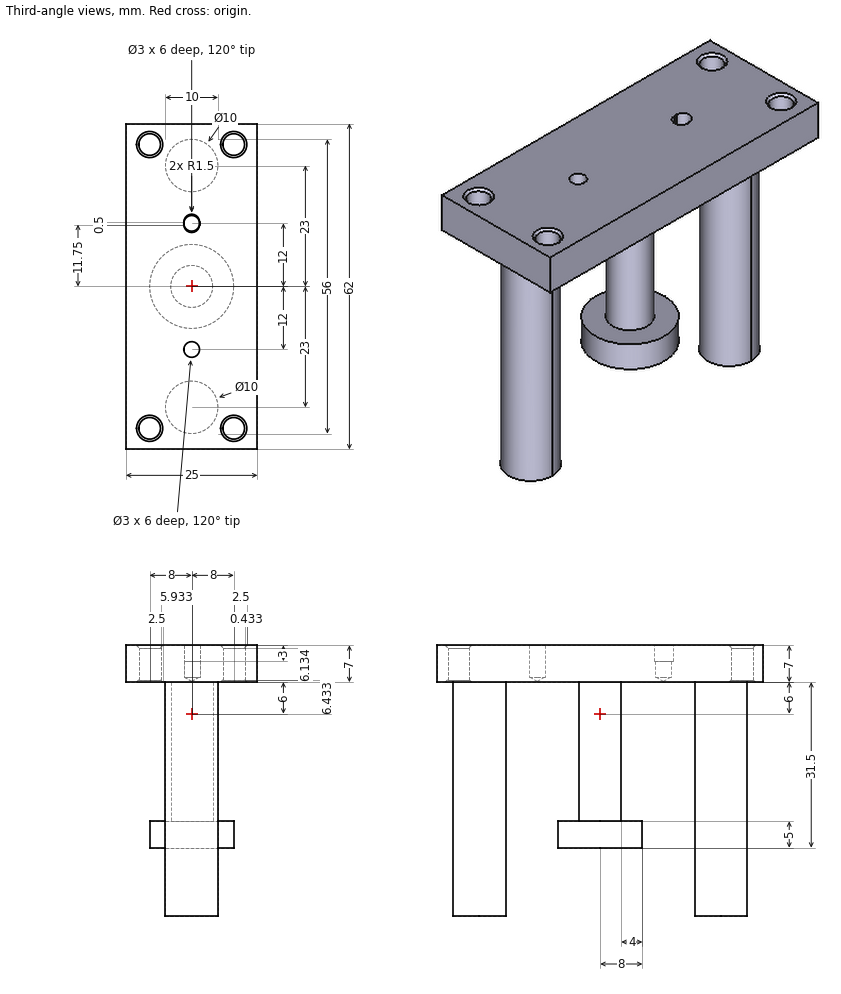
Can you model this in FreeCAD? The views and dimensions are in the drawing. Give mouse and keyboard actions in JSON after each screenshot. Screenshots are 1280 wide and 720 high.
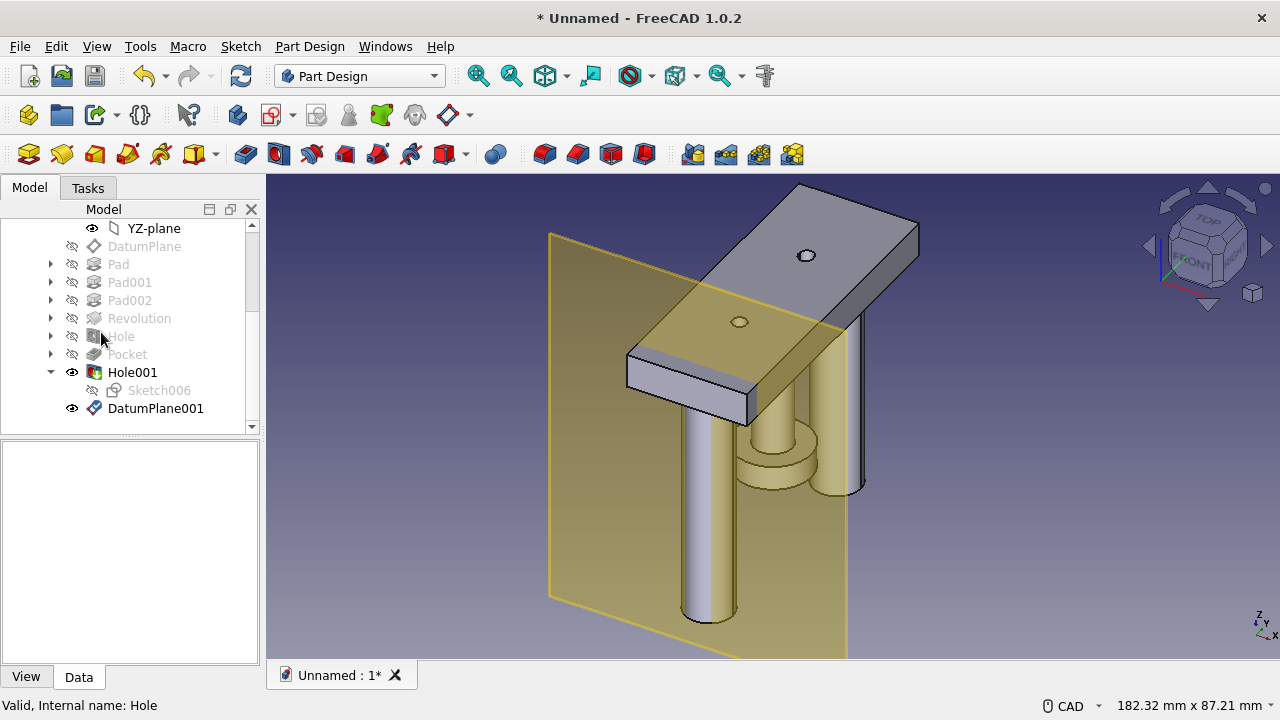
{"action": "left_click", "coordinate": [117, 408]}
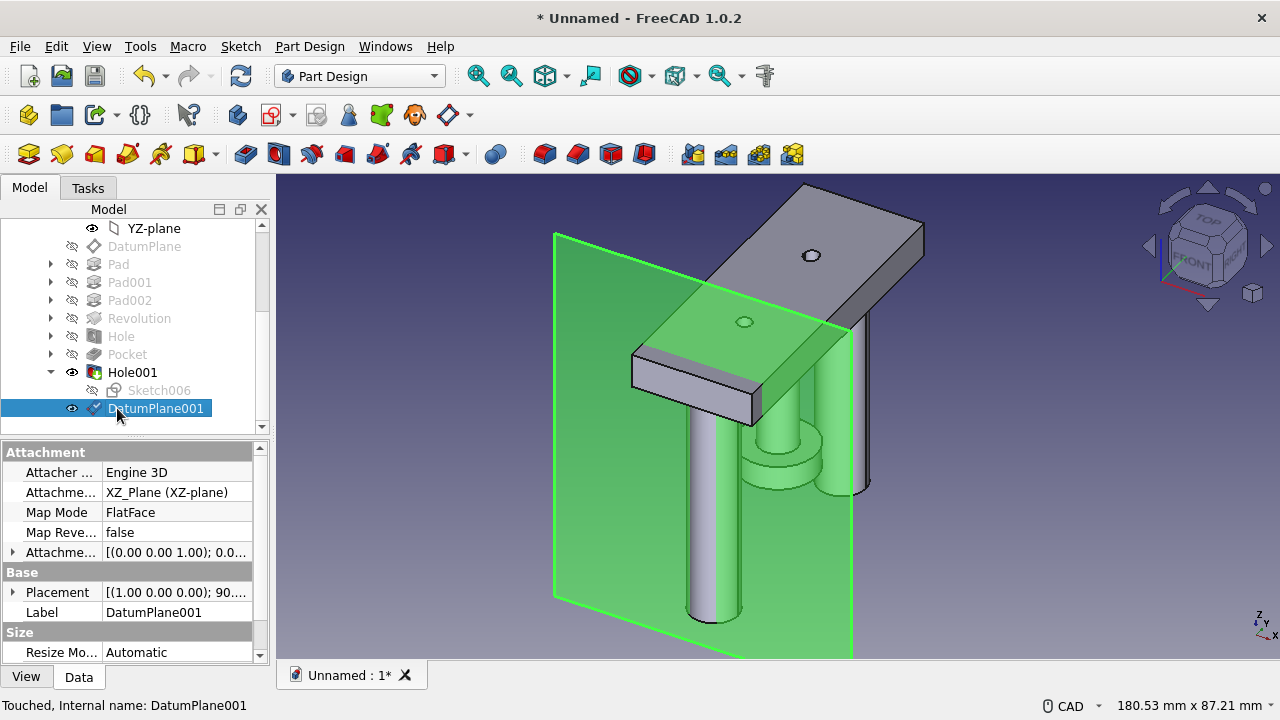
{"action": "left_click", "coordinate": [270, 116]}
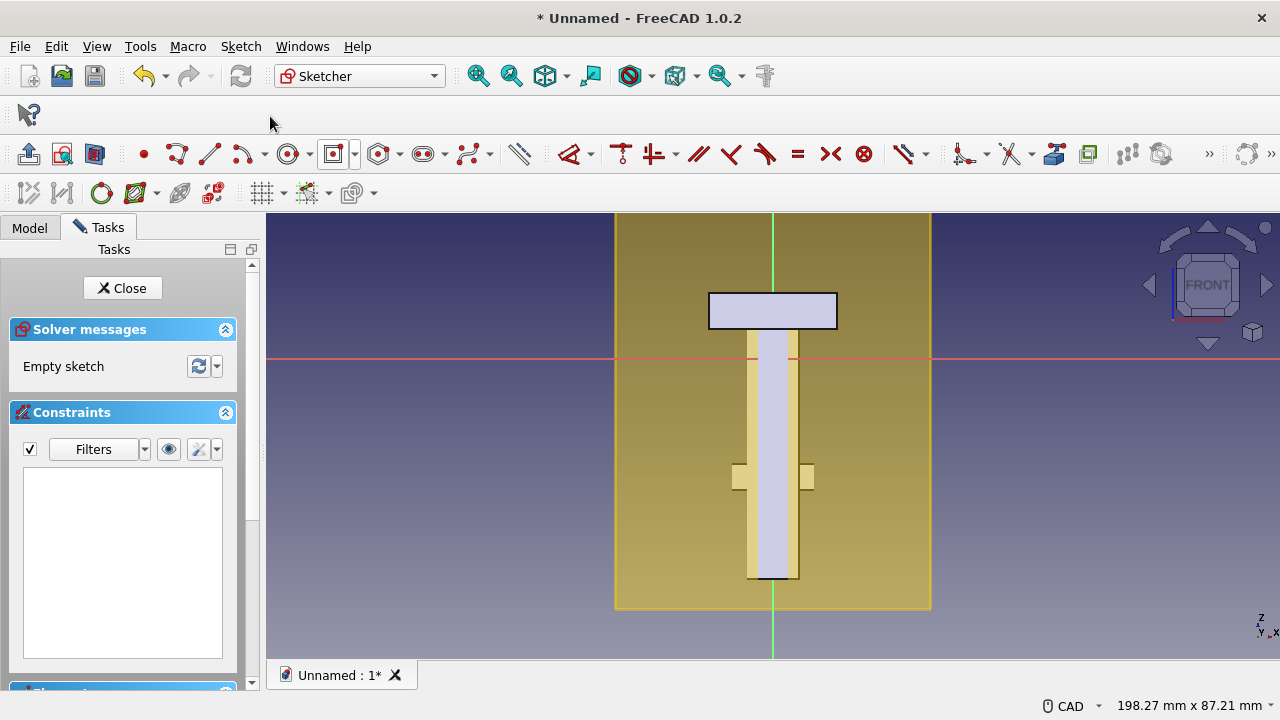
{"action": "left_click", "coordinate": [95, 154]}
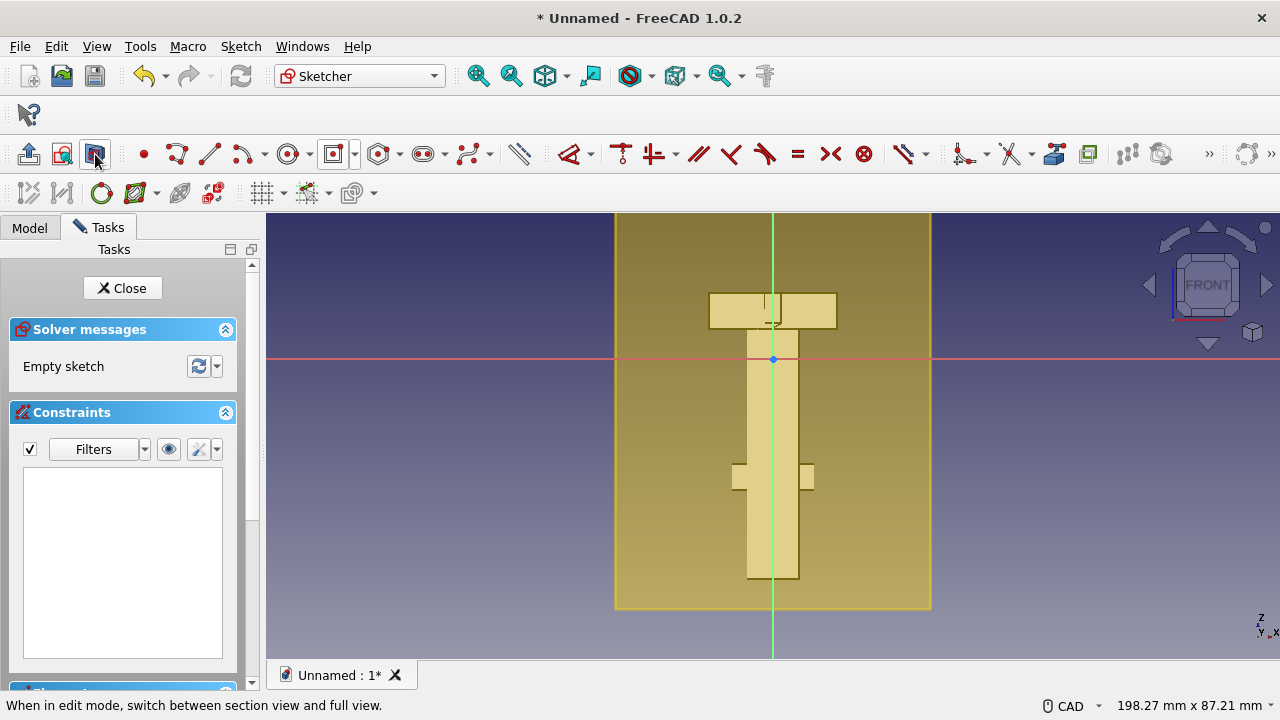
{"action": "scroll", "coordinate": [831, 290], "scroll_direction": "up", "scroll_amount": 7}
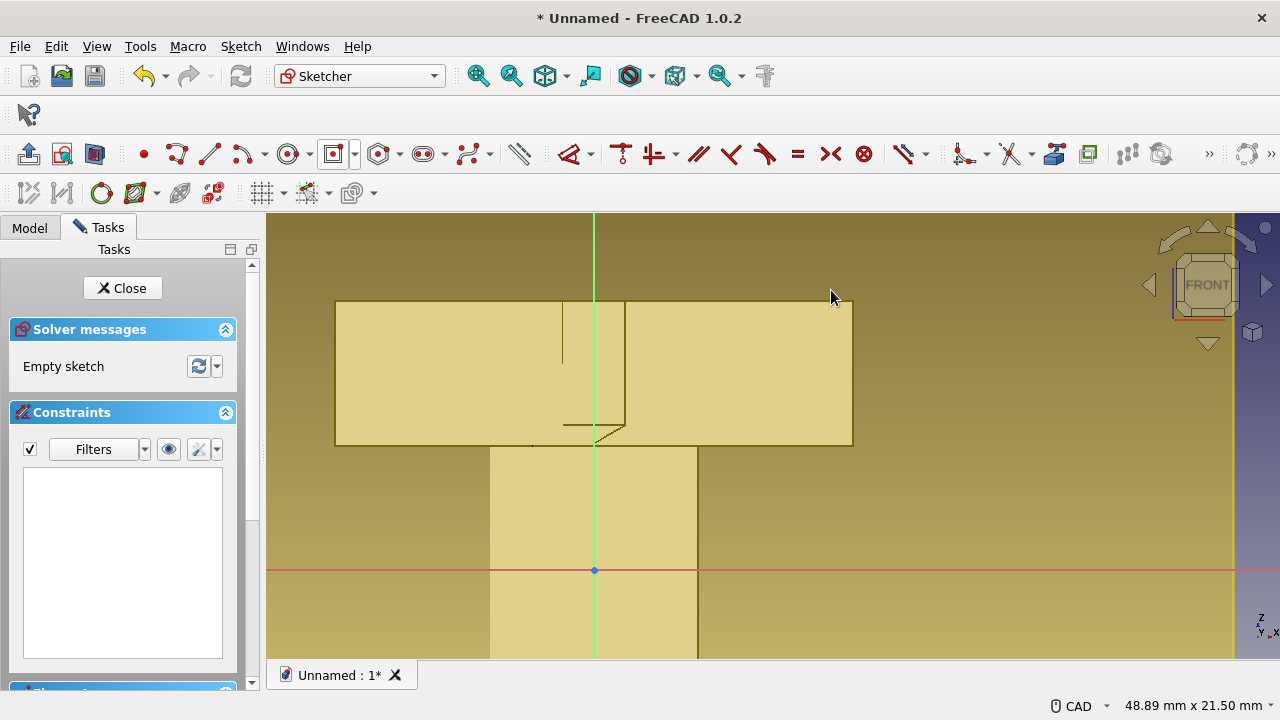
{"action": "left_click", "coordinate": [177, 154]}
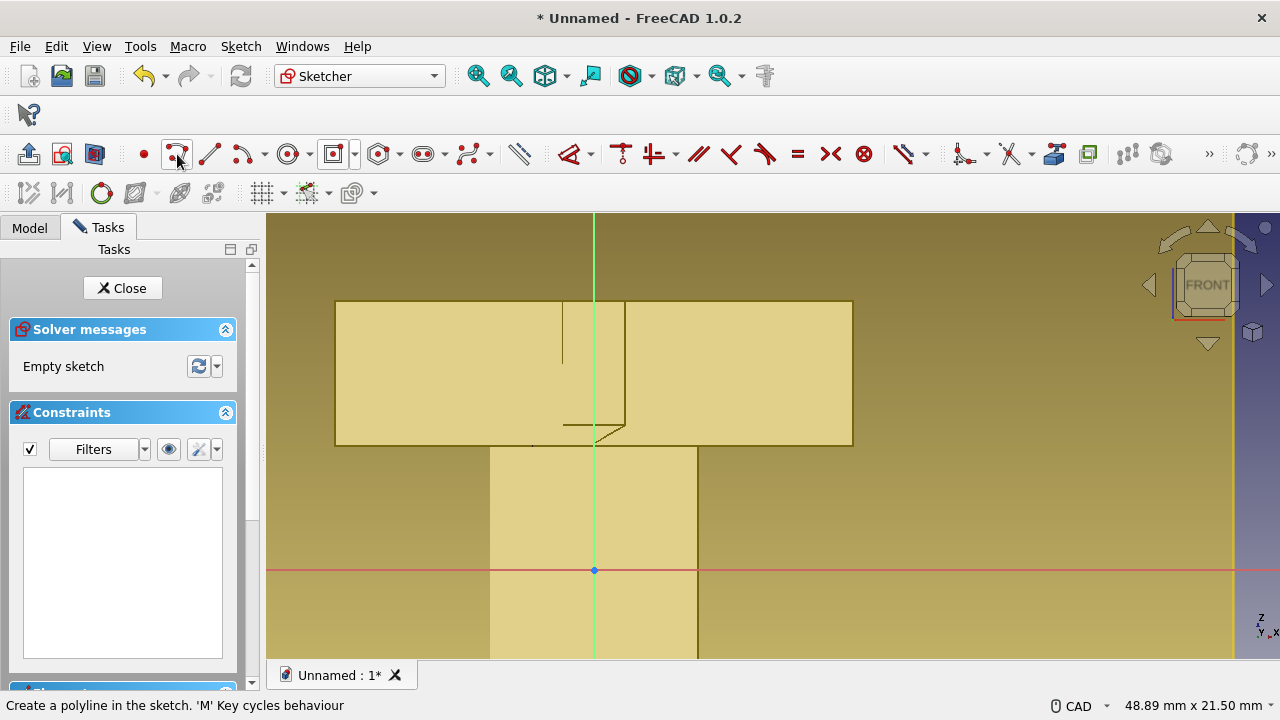
{"action": "left_click", "coordinate": [760, 446]}
{"action": "left_click", "coordinate": [760, 301]}
{"action": "left_click", "coordinate": [812, 301]}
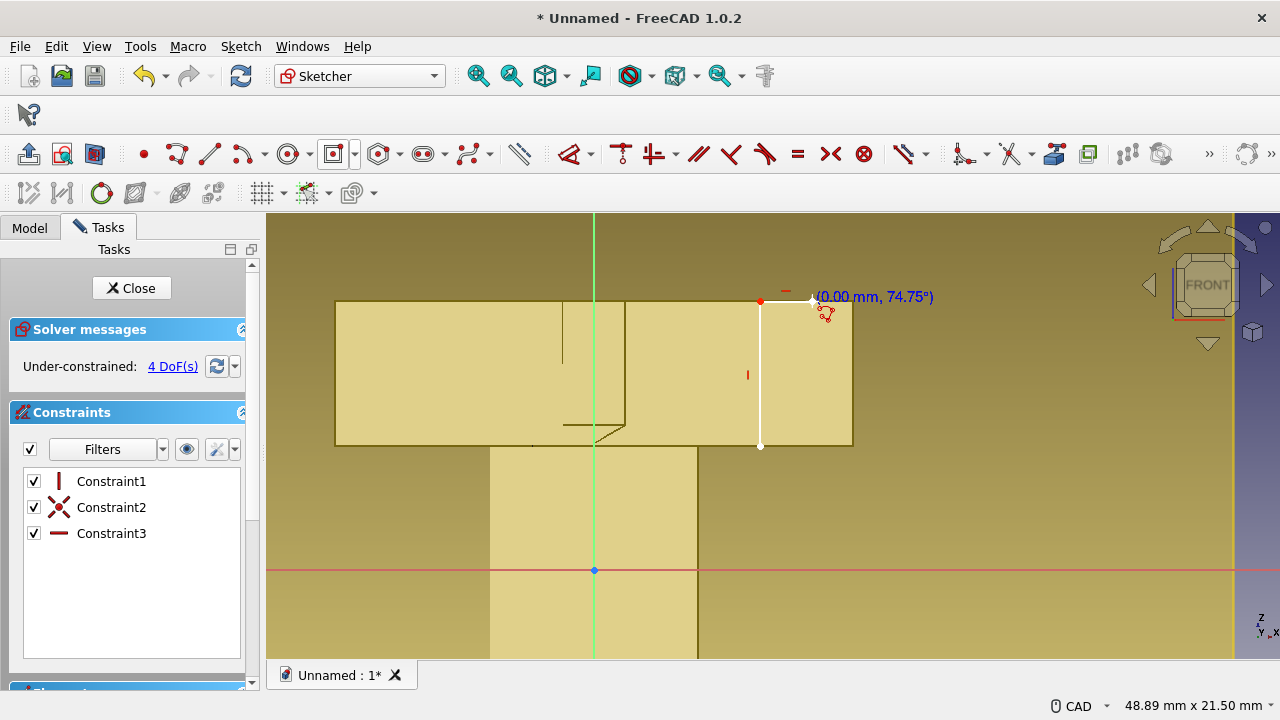
{"action": "scroll", "coordinate": [803, 310], "scroll_direction": "up", "scroll_amount": 3}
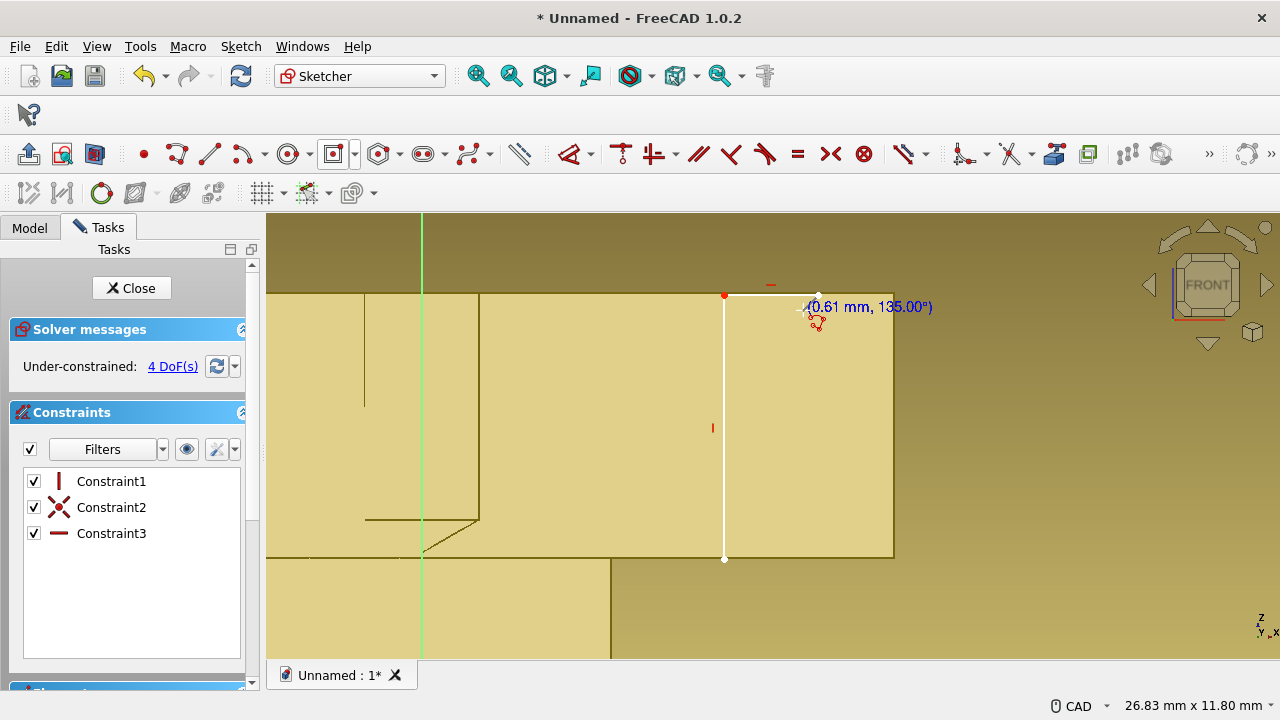
{"action": "left_click", "coordinate": [802, 309]}
{"action": "left_click", "coordinate": [802, 541]}
{"action": "left_click", "coordinate": [819, 558]}
{"action": "left_click", "coordinate": [724, 559]}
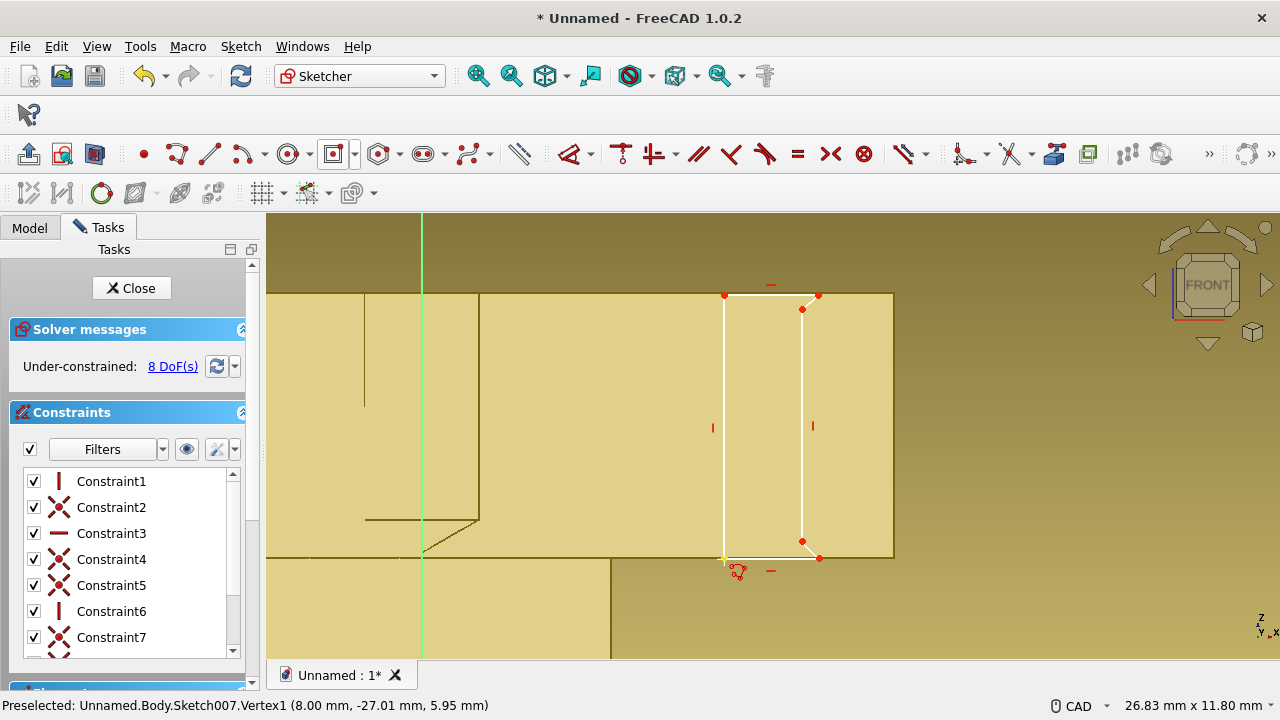
{"action": "left_click", "coordinate": [210, 154]}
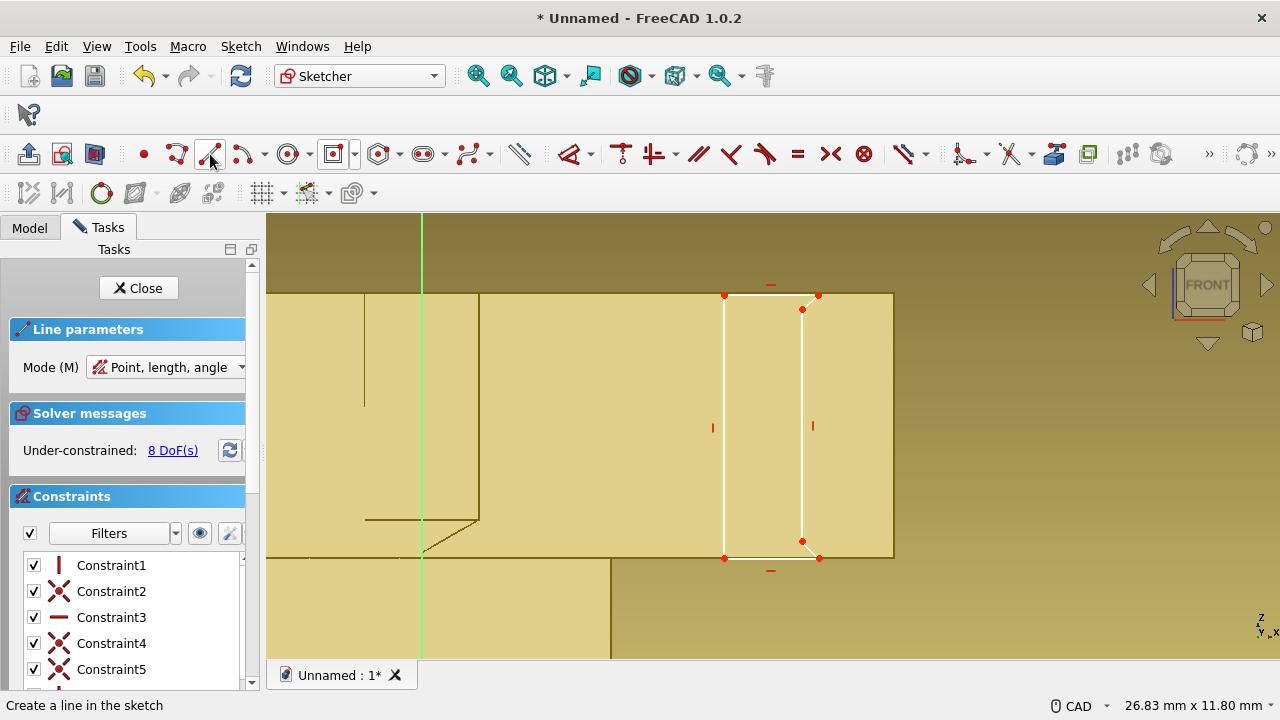
{"action": "left_click", "coordinate": [724, 584]}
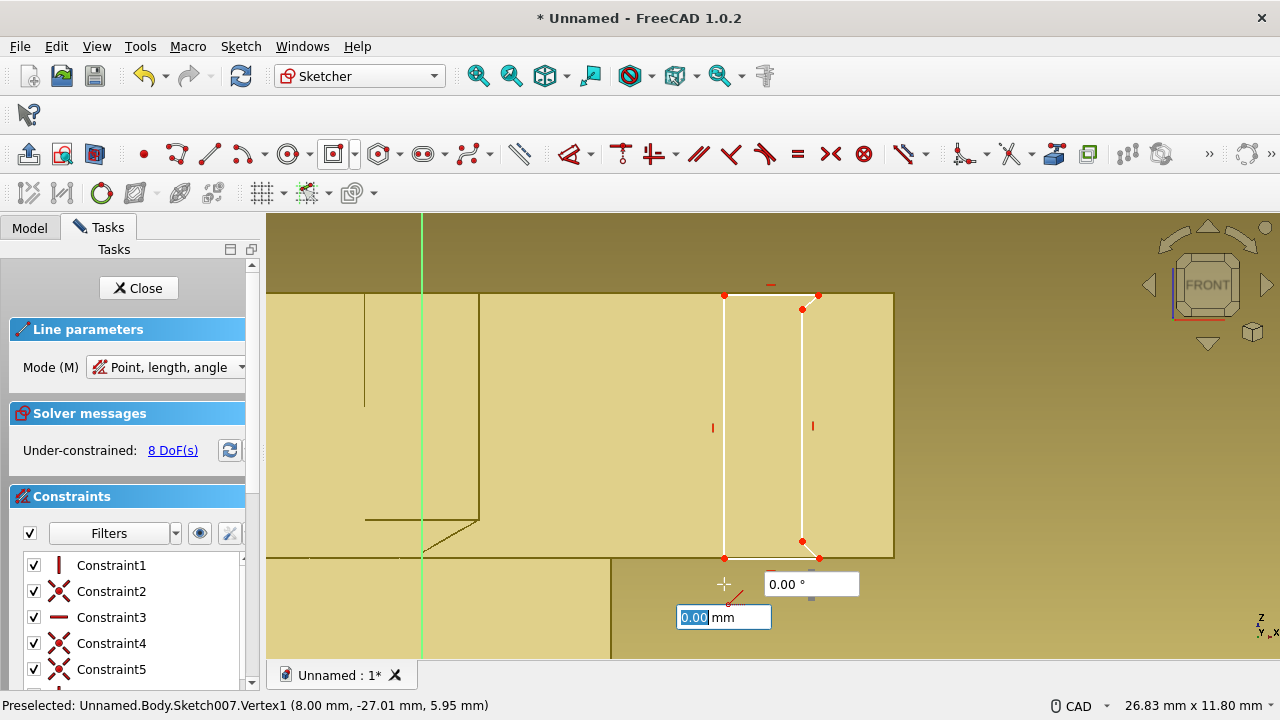
{"action": "scroll", "coordinate": [807, 311], "scroll_direction": "down", "scroll_amount": 3}